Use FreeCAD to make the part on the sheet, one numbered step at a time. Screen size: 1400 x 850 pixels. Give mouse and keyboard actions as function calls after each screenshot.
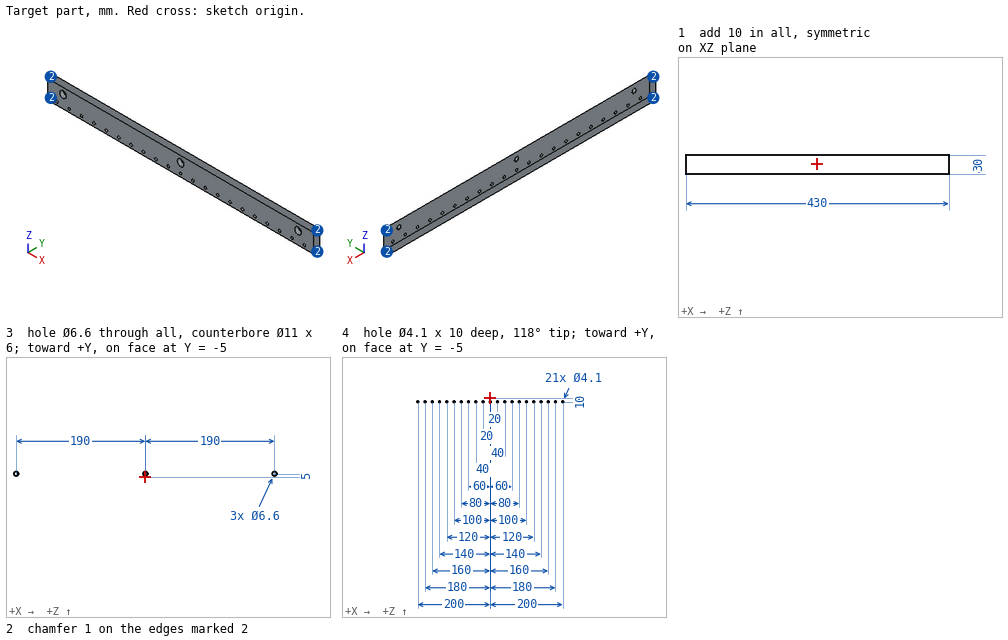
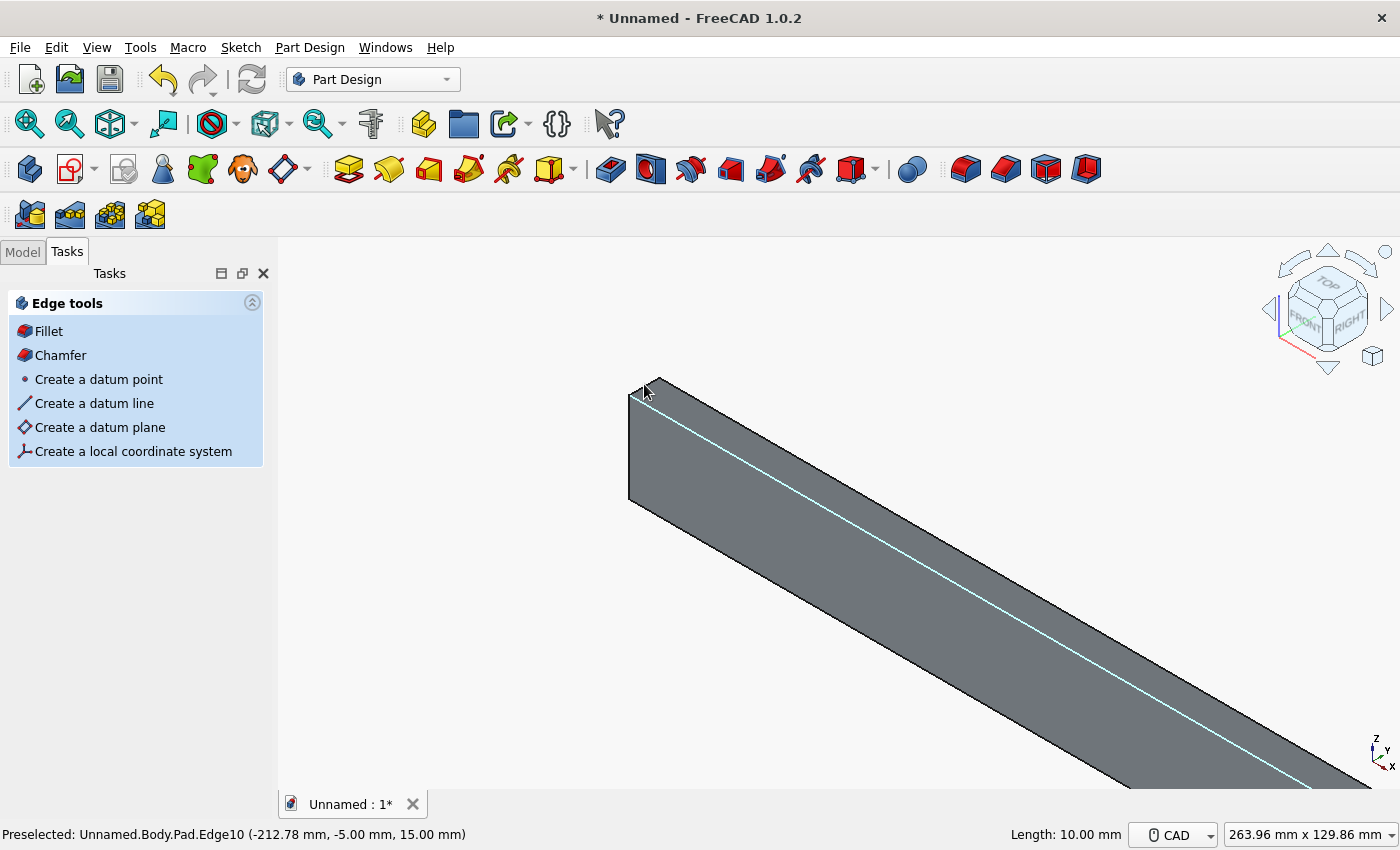
key(v)
key(f)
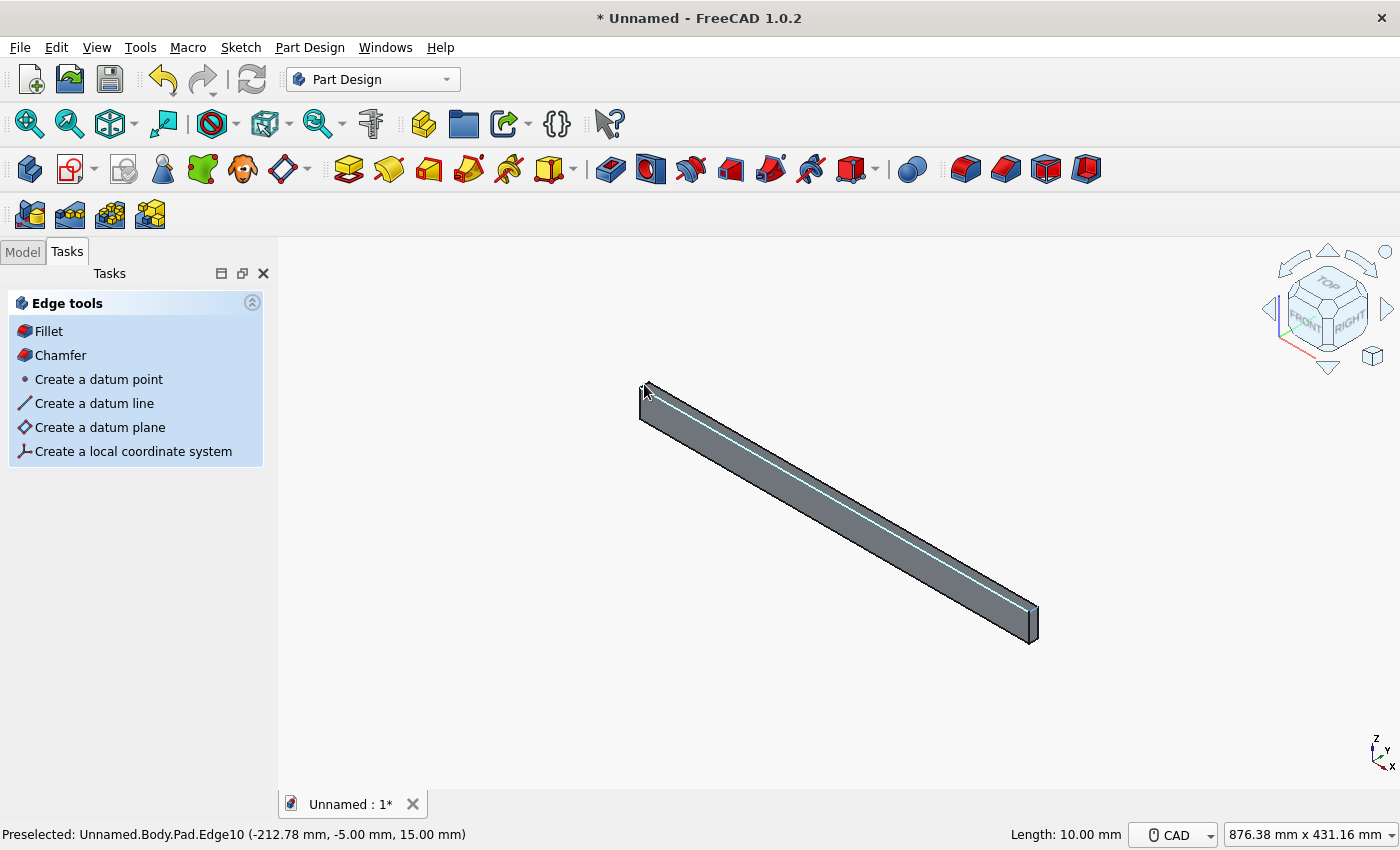
key(2)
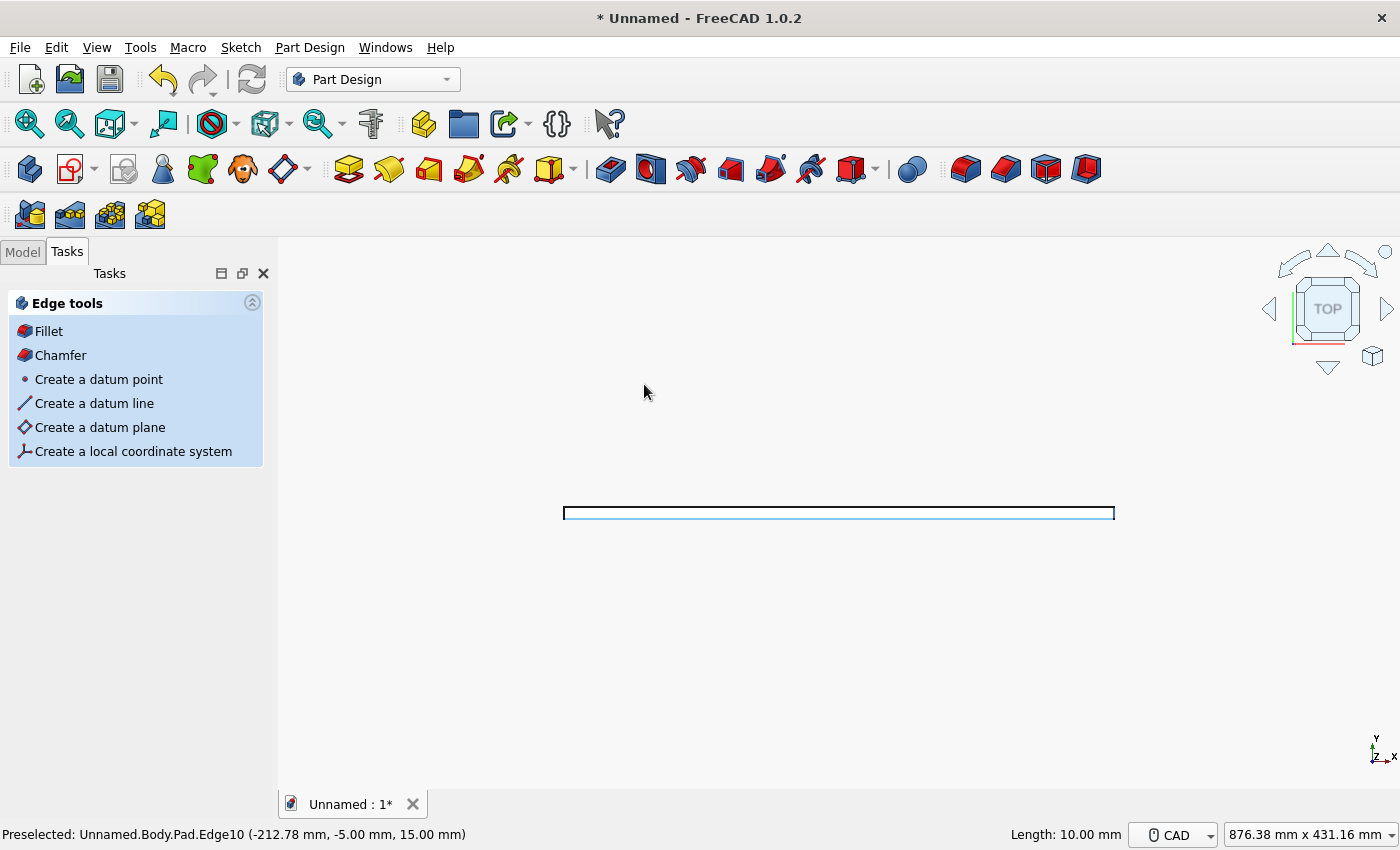
click(564, 512, ctrl)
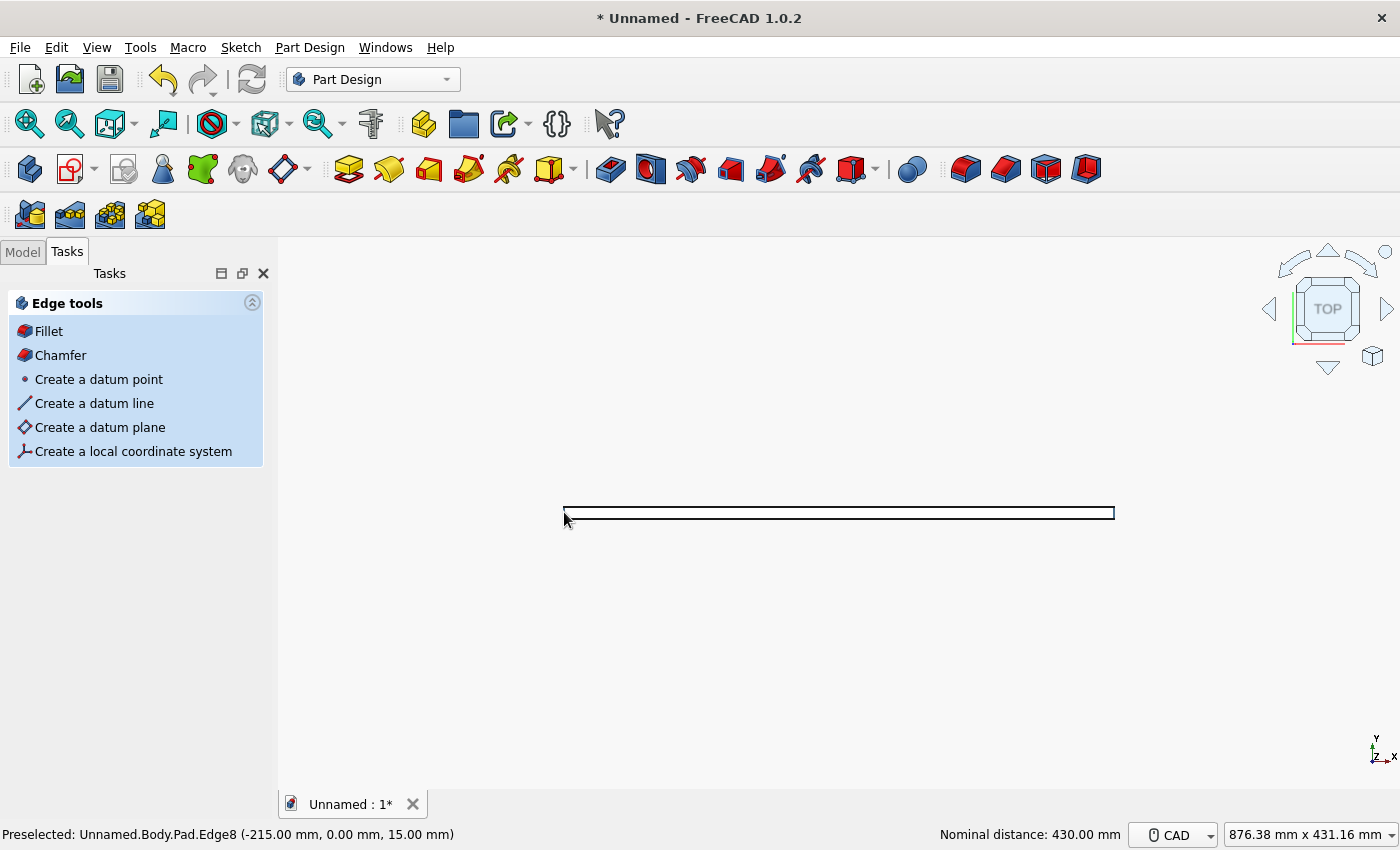
scroll(564, 512, up, 6)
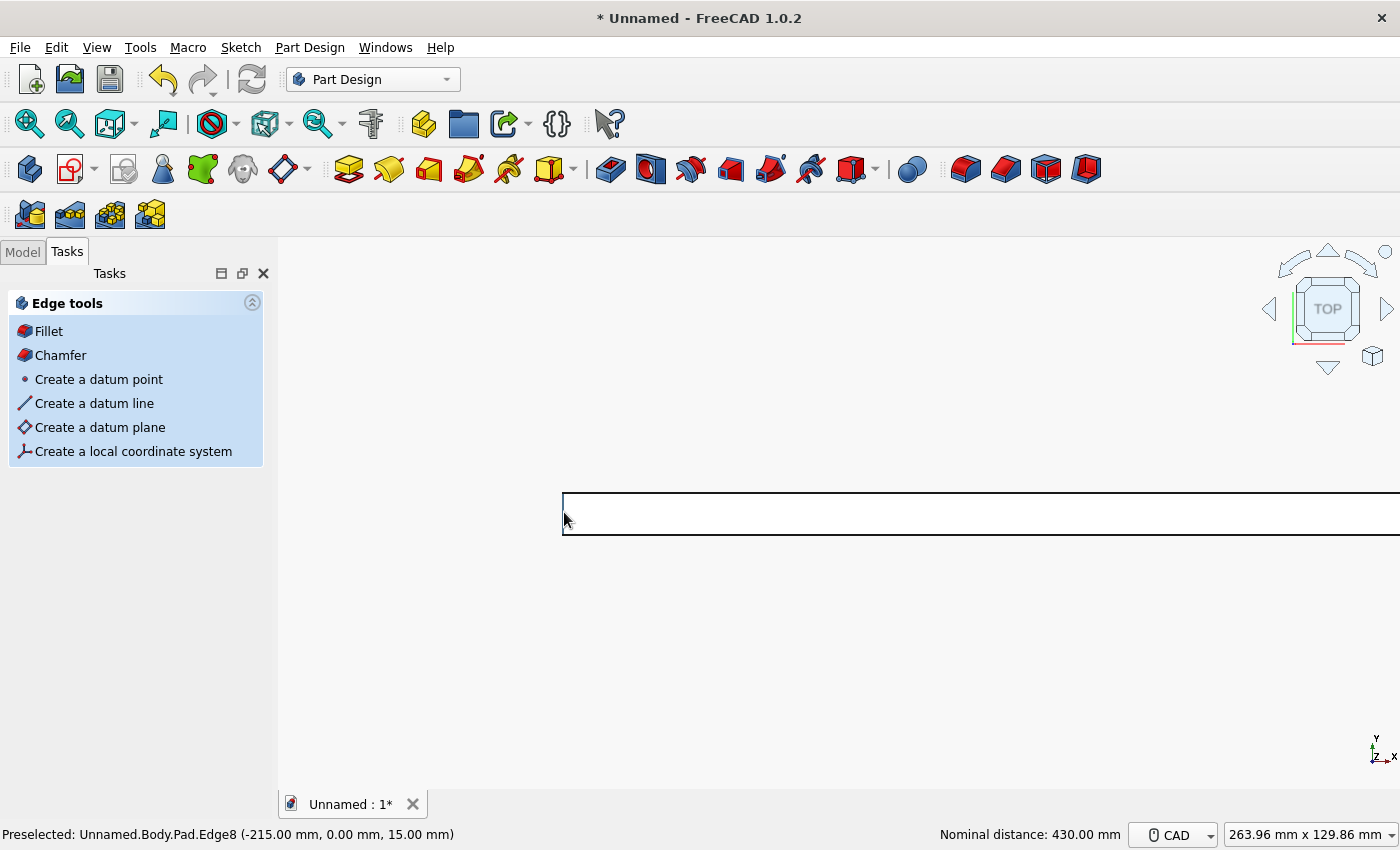
key(v)
key(f)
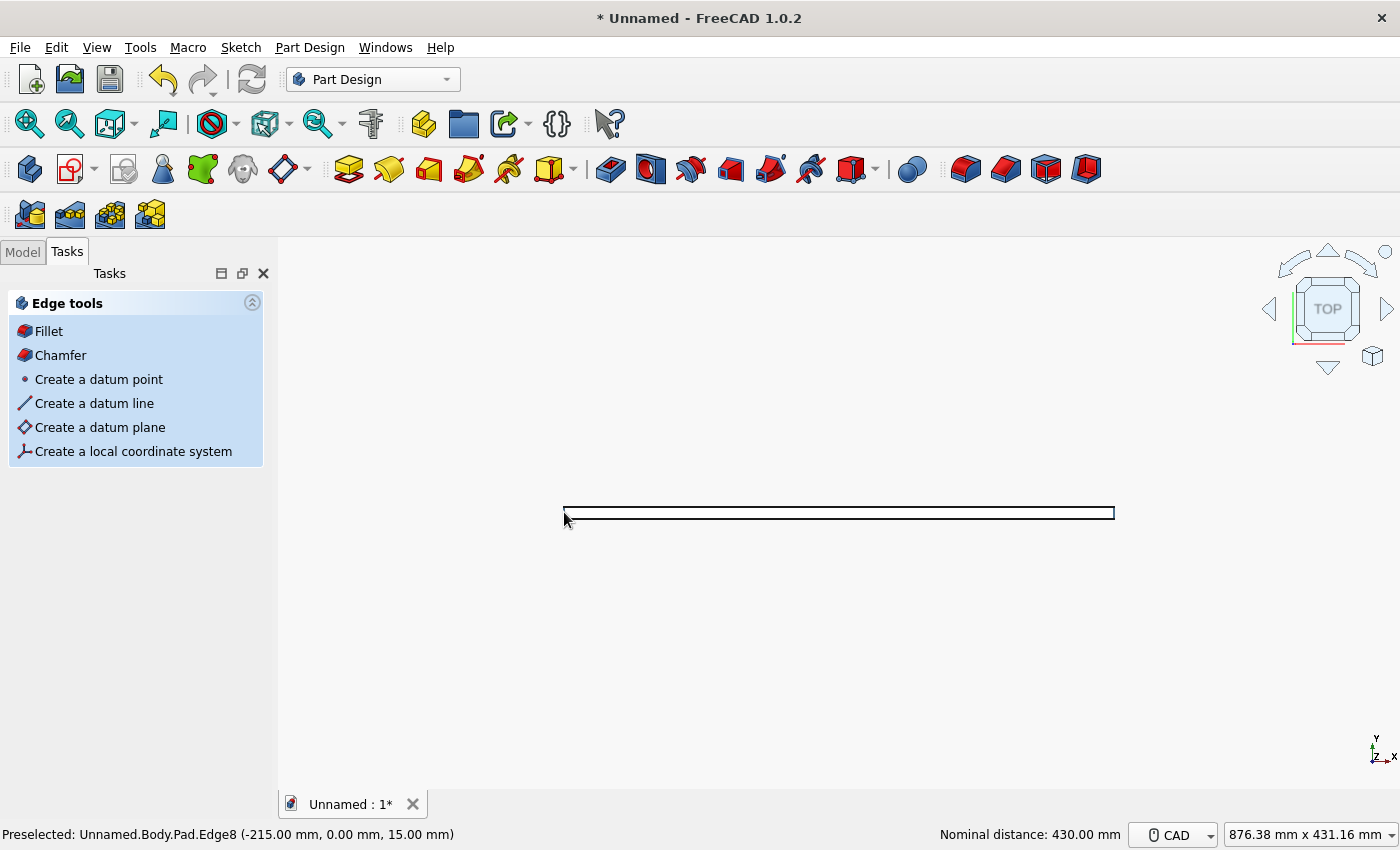
key(1)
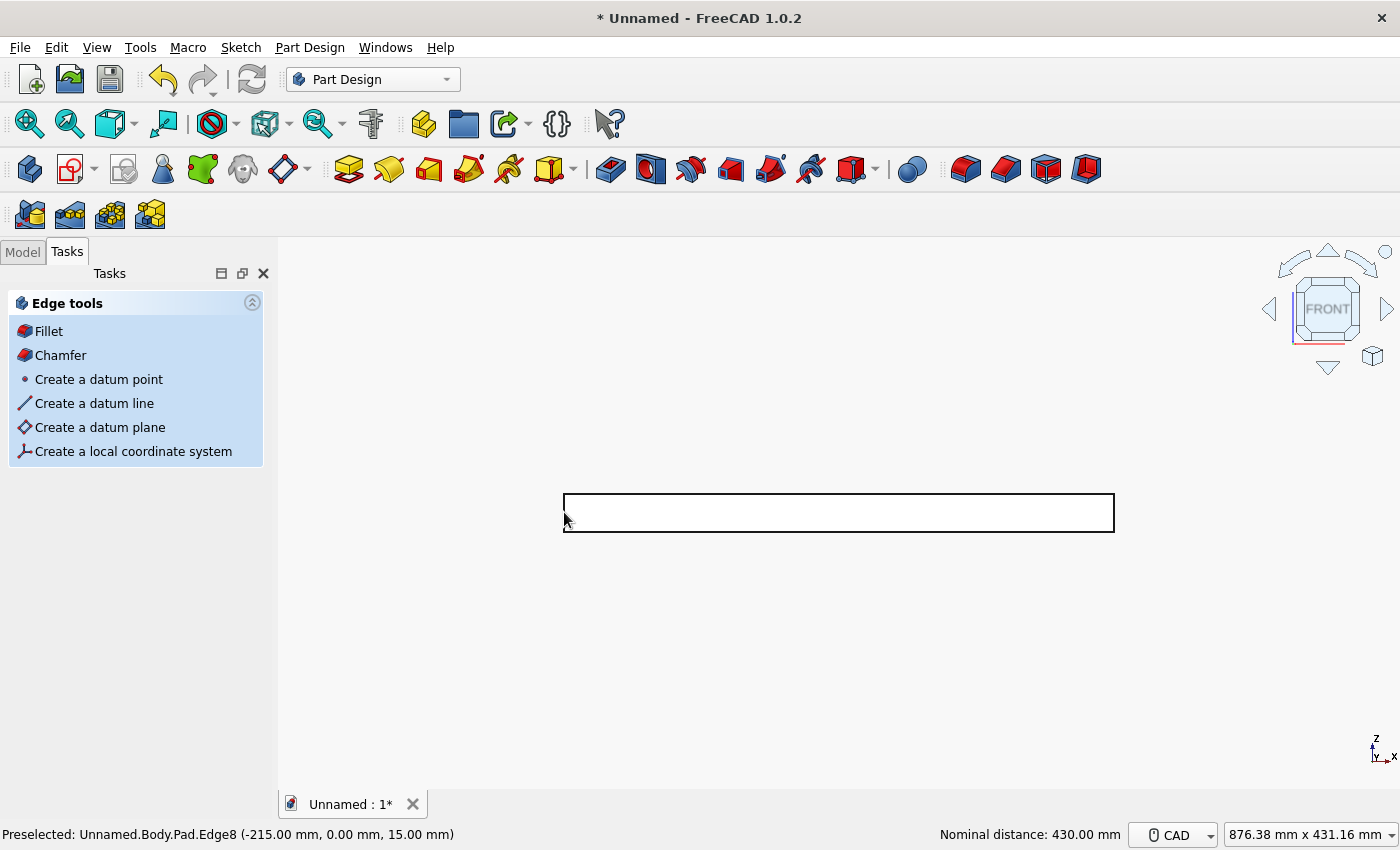
scroll(564, 531, up, 6)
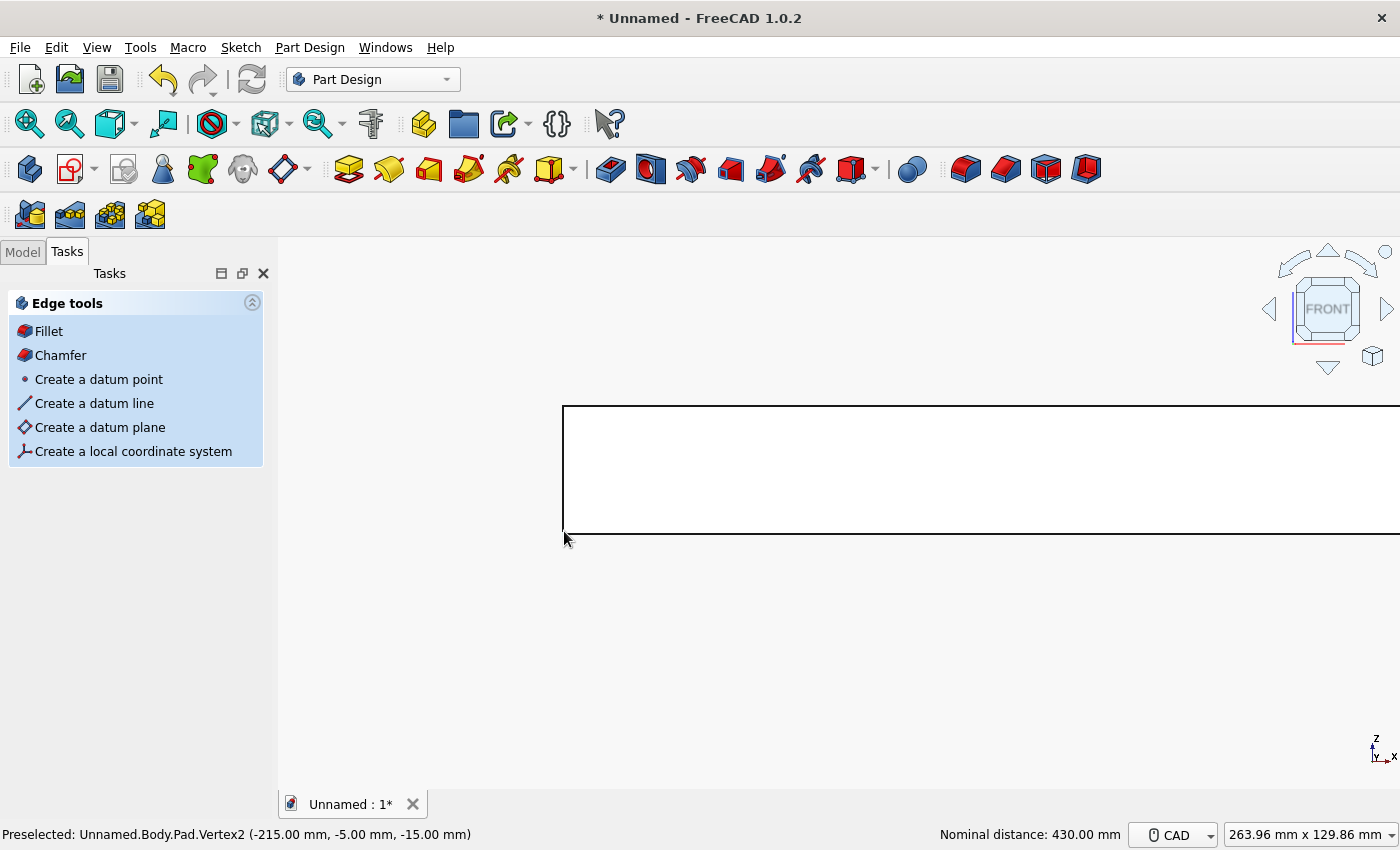
click(30, 124)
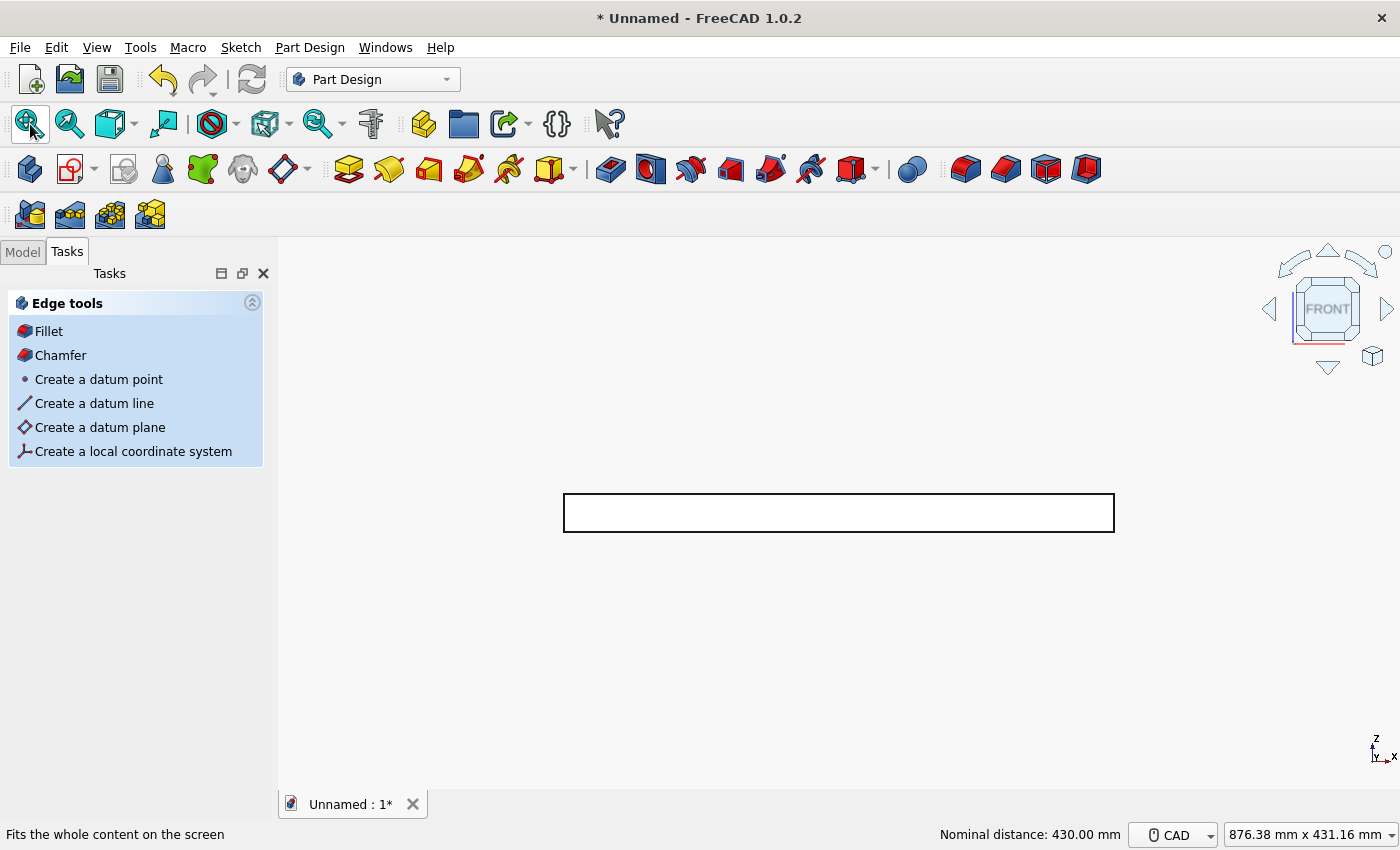
key(3)